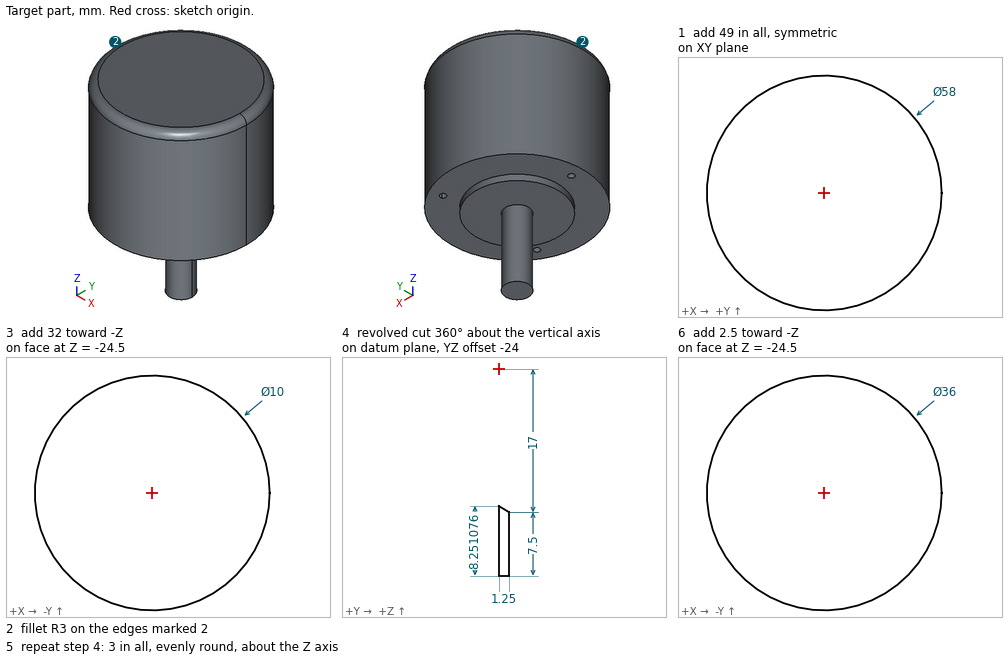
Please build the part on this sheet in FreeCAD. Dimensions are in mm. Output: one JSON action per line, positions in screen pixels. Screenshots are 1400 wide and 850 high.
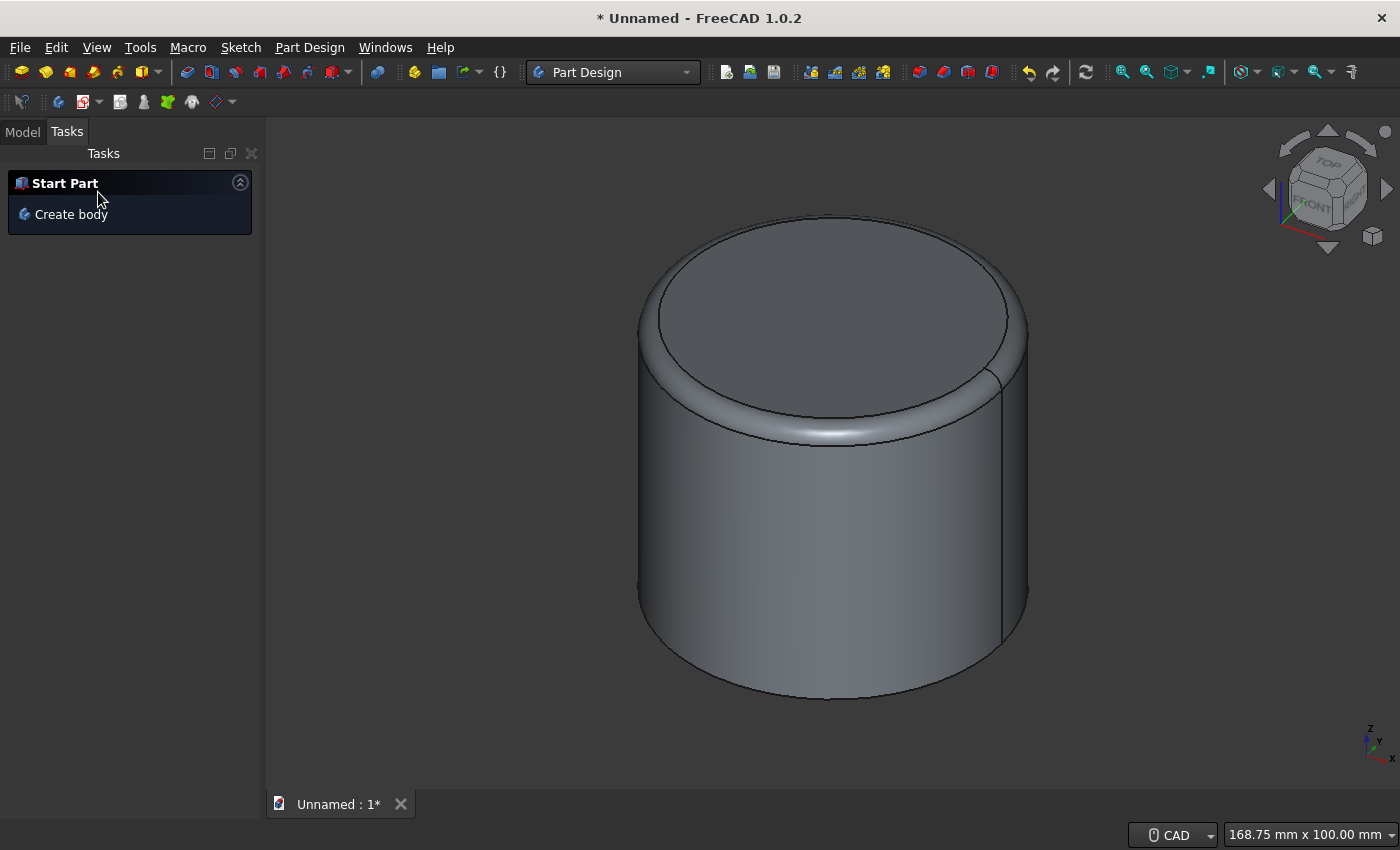
{"action": "key", "text": "5"}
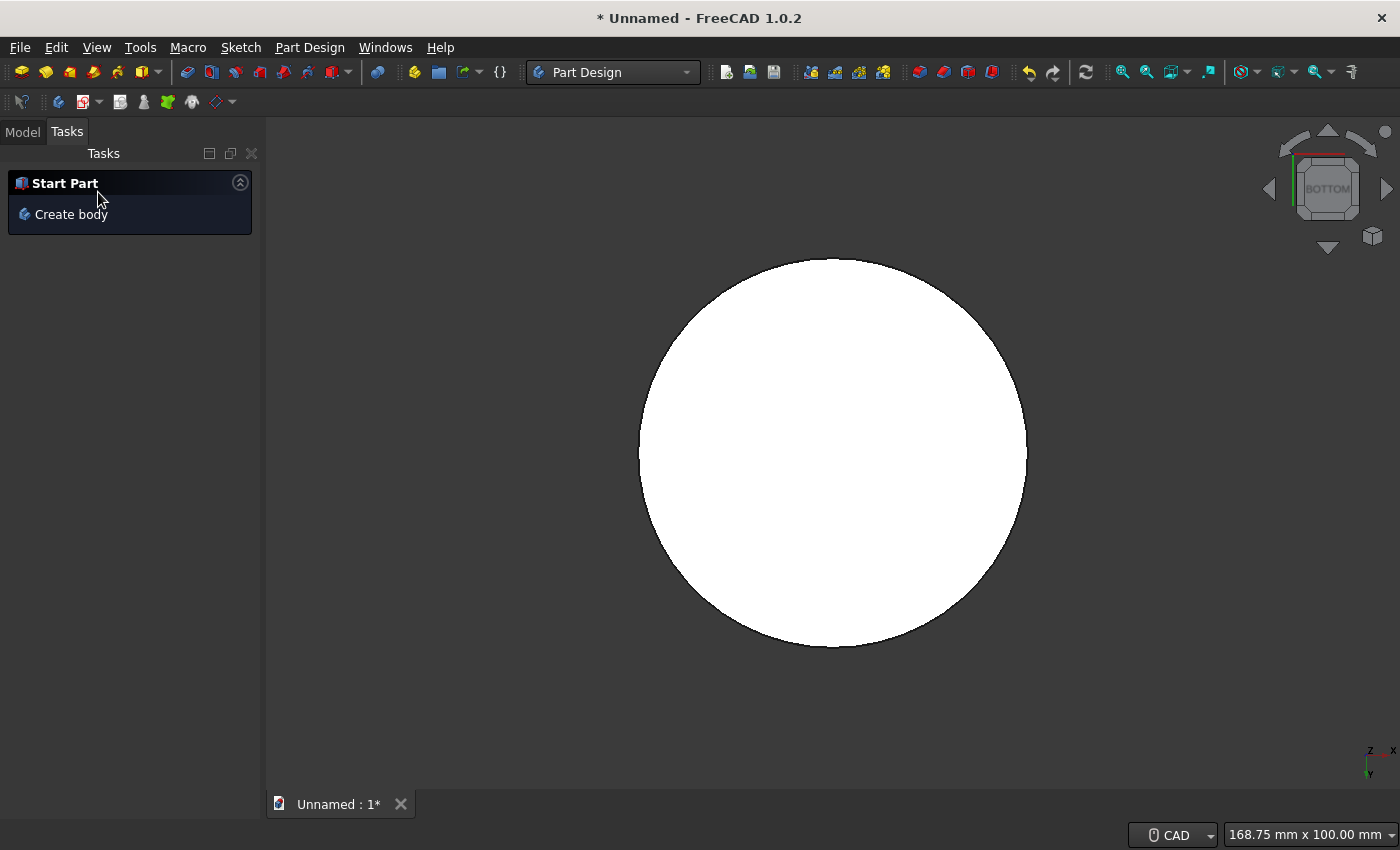
{"action": "left_click", "coordinate": [833, 452]}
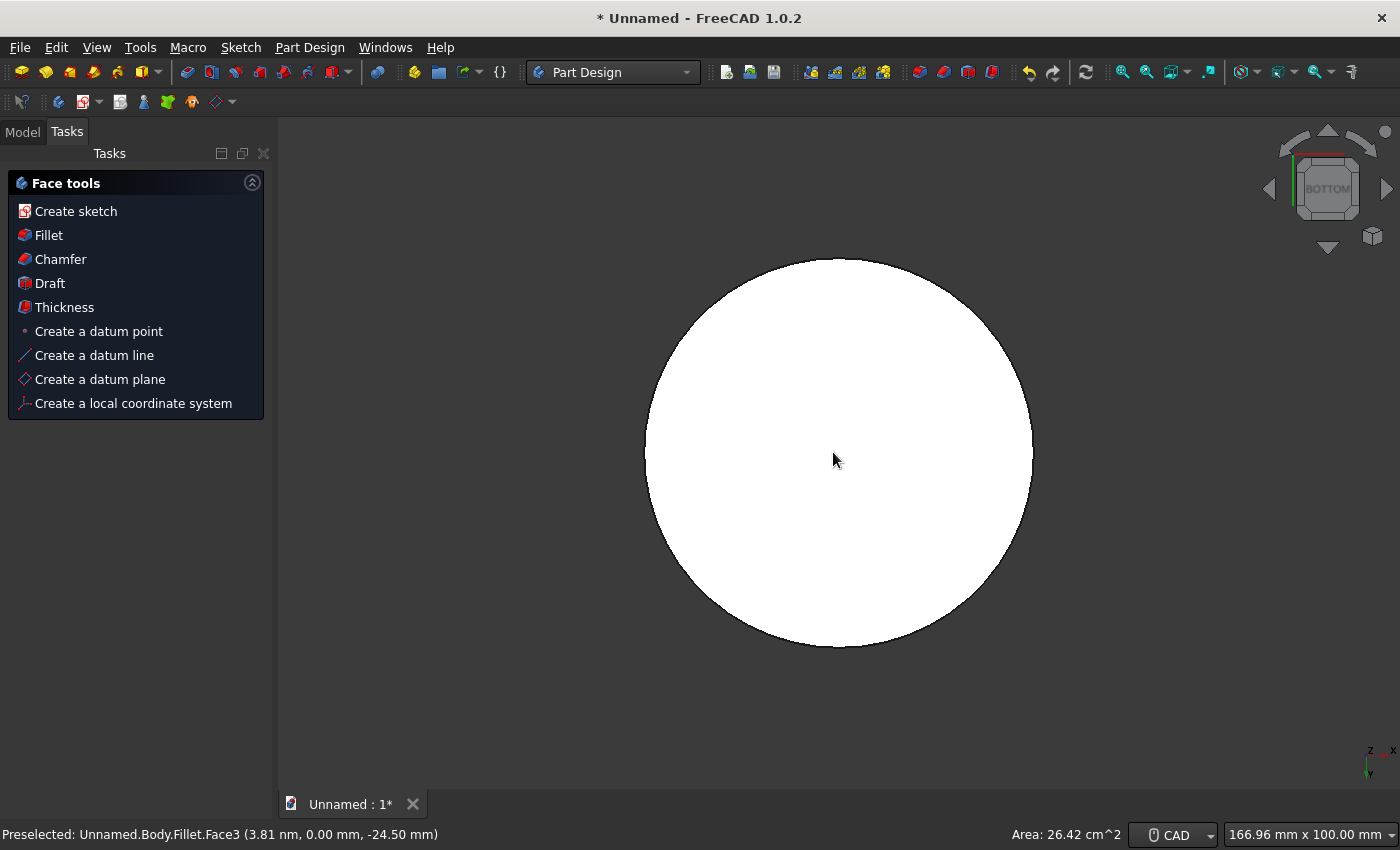
{"action": "left_click", "coordinate": [84, 102]}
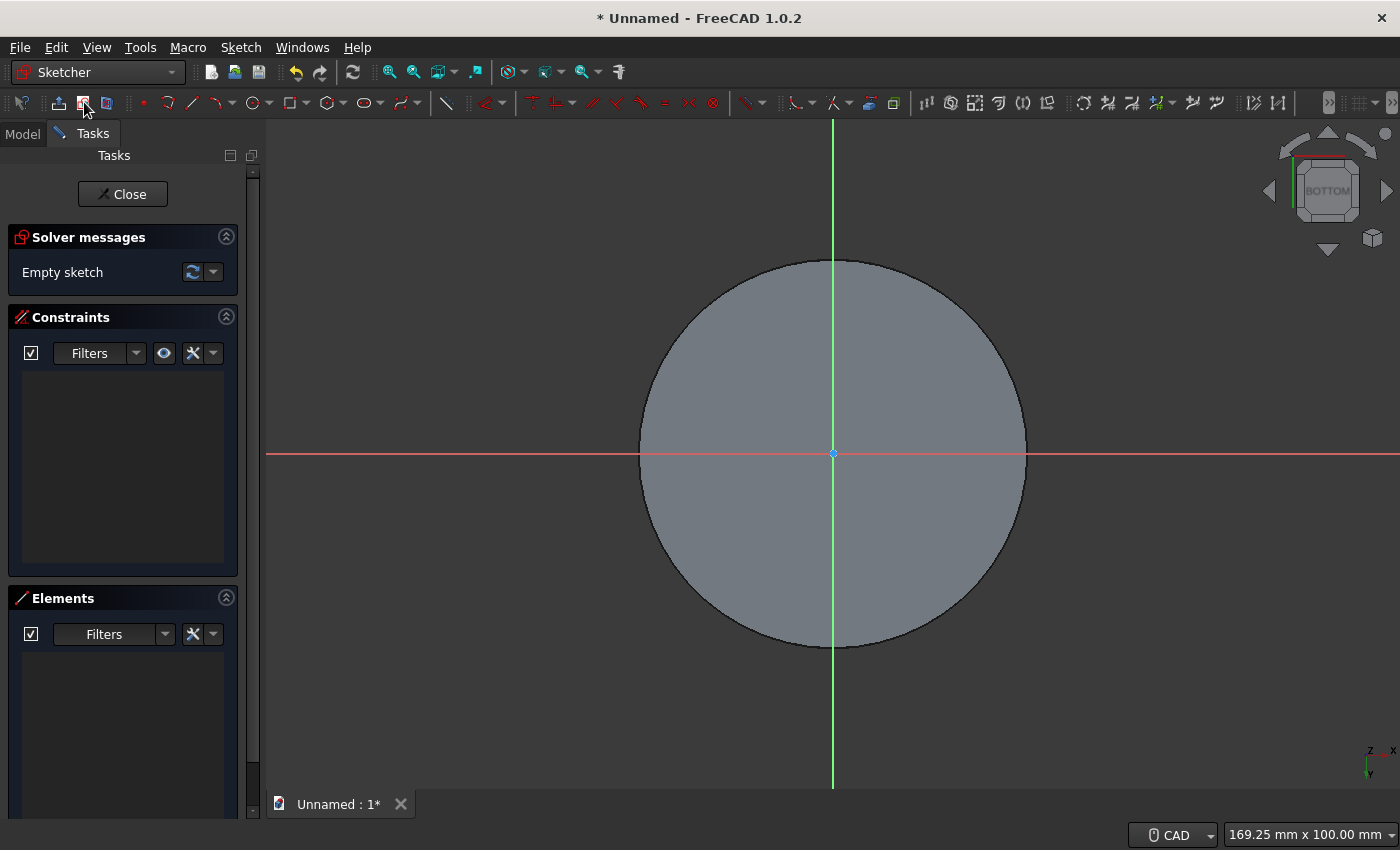
{"action": "scroll", "coordinate": [847, 454], "scroll_direction": "up", "scroll_amount": 9}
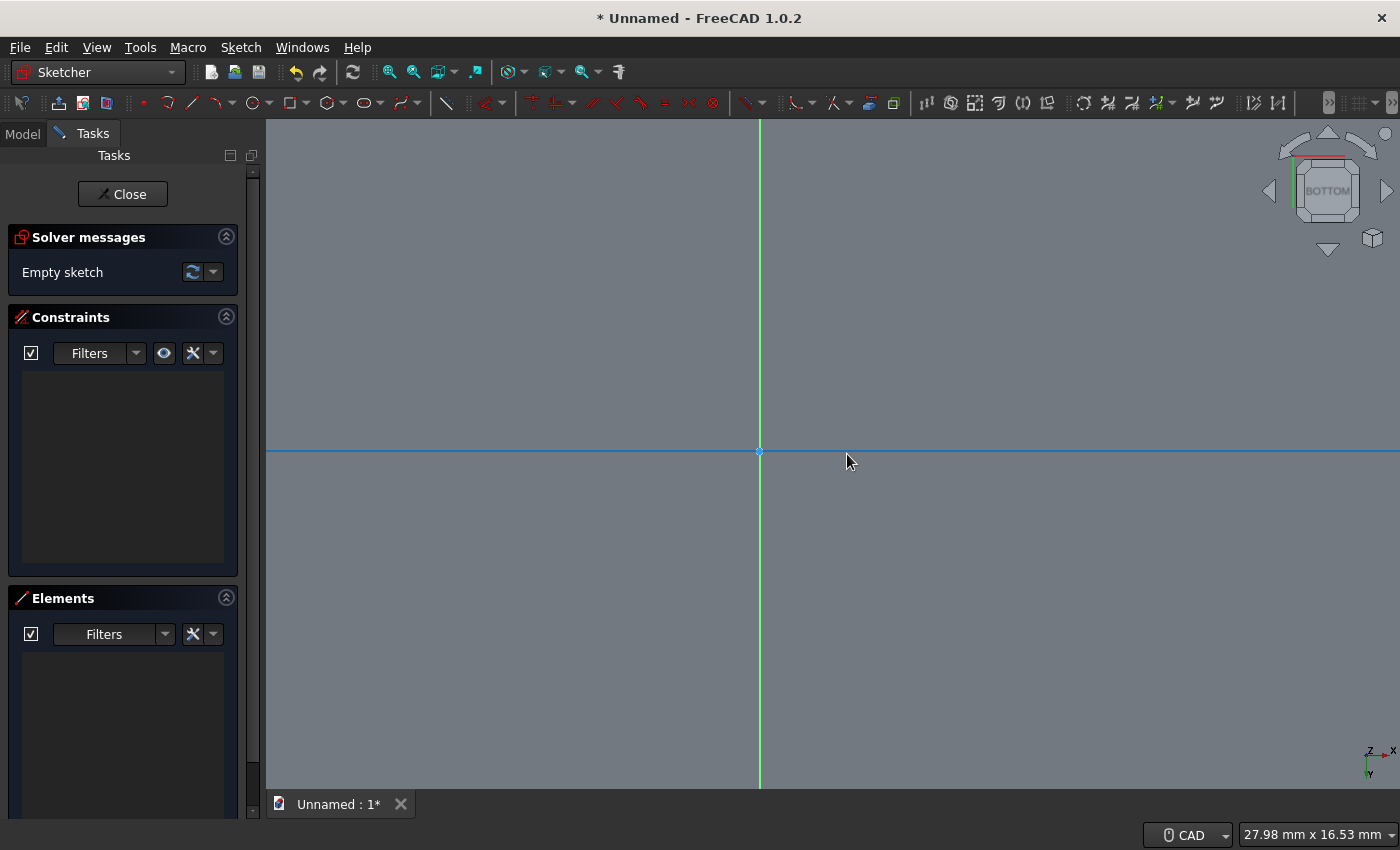
{"action": "left_click", "coordinate": [254, 104]}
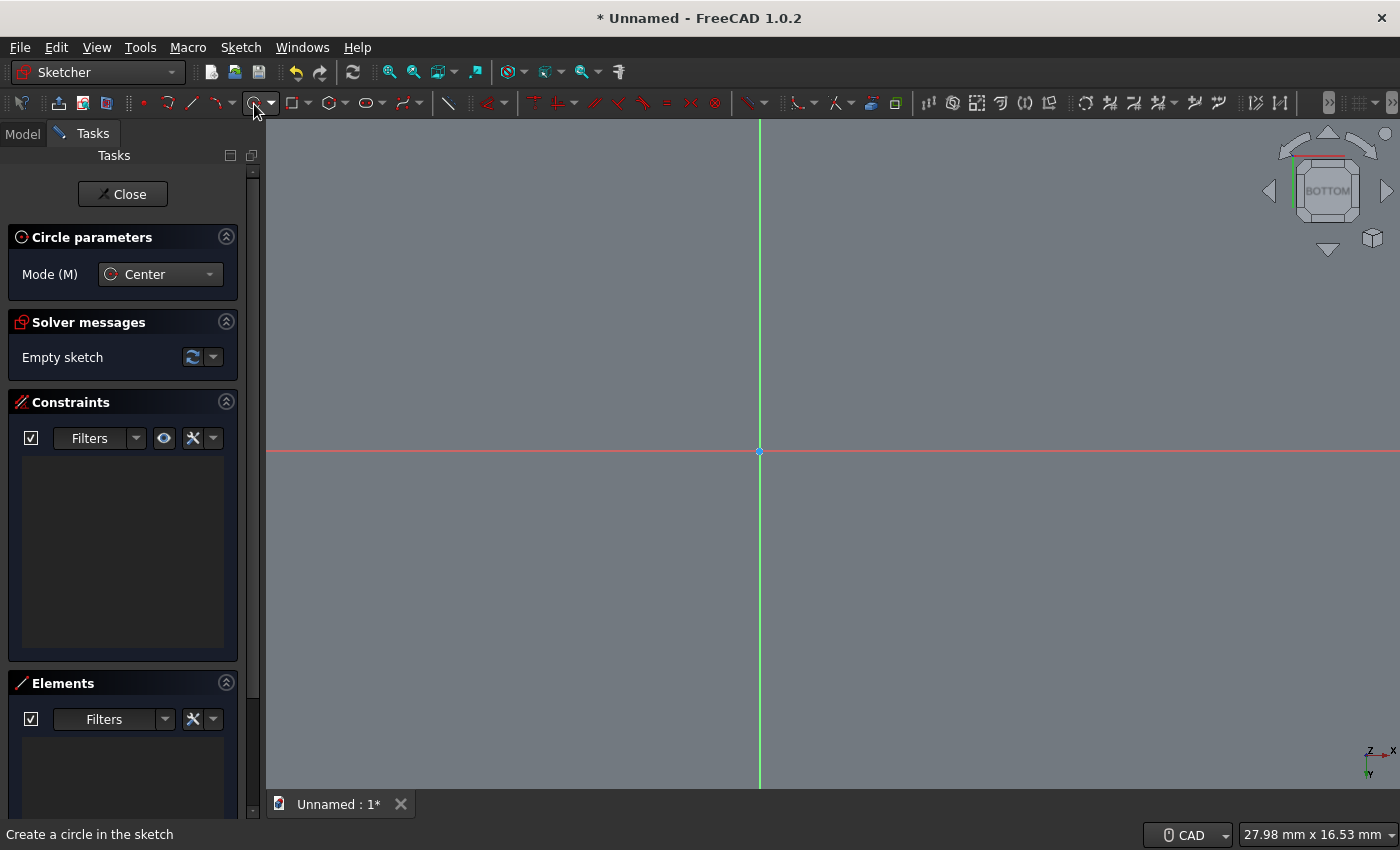
{"action": "left_click", "coordinate": [760, 451]}
{"action": "left_click", "coordinate": [903, 308]}
{"action": "key", "text": "Escape"}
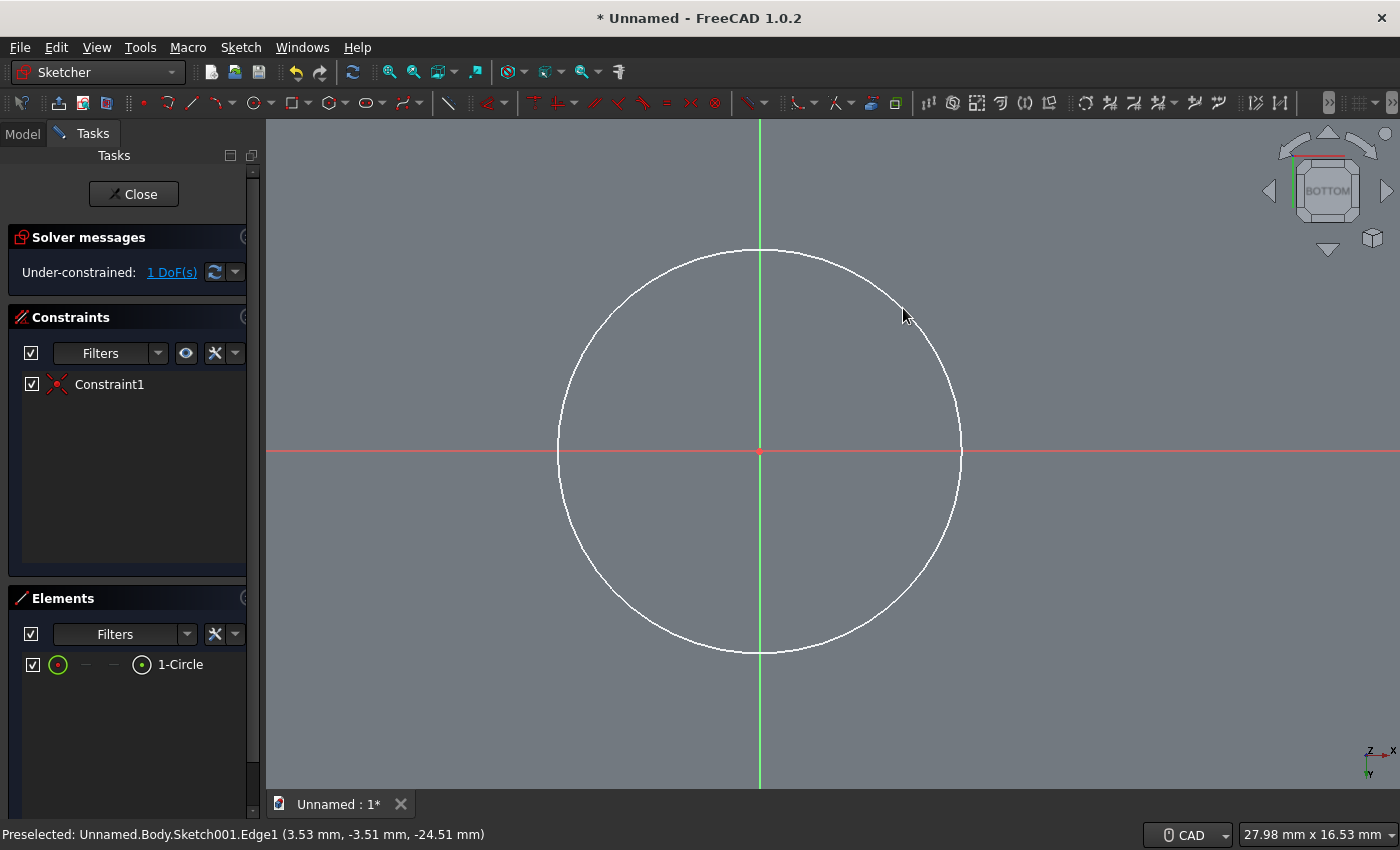
{"action": "left_click", "coordinate": [488, 104]}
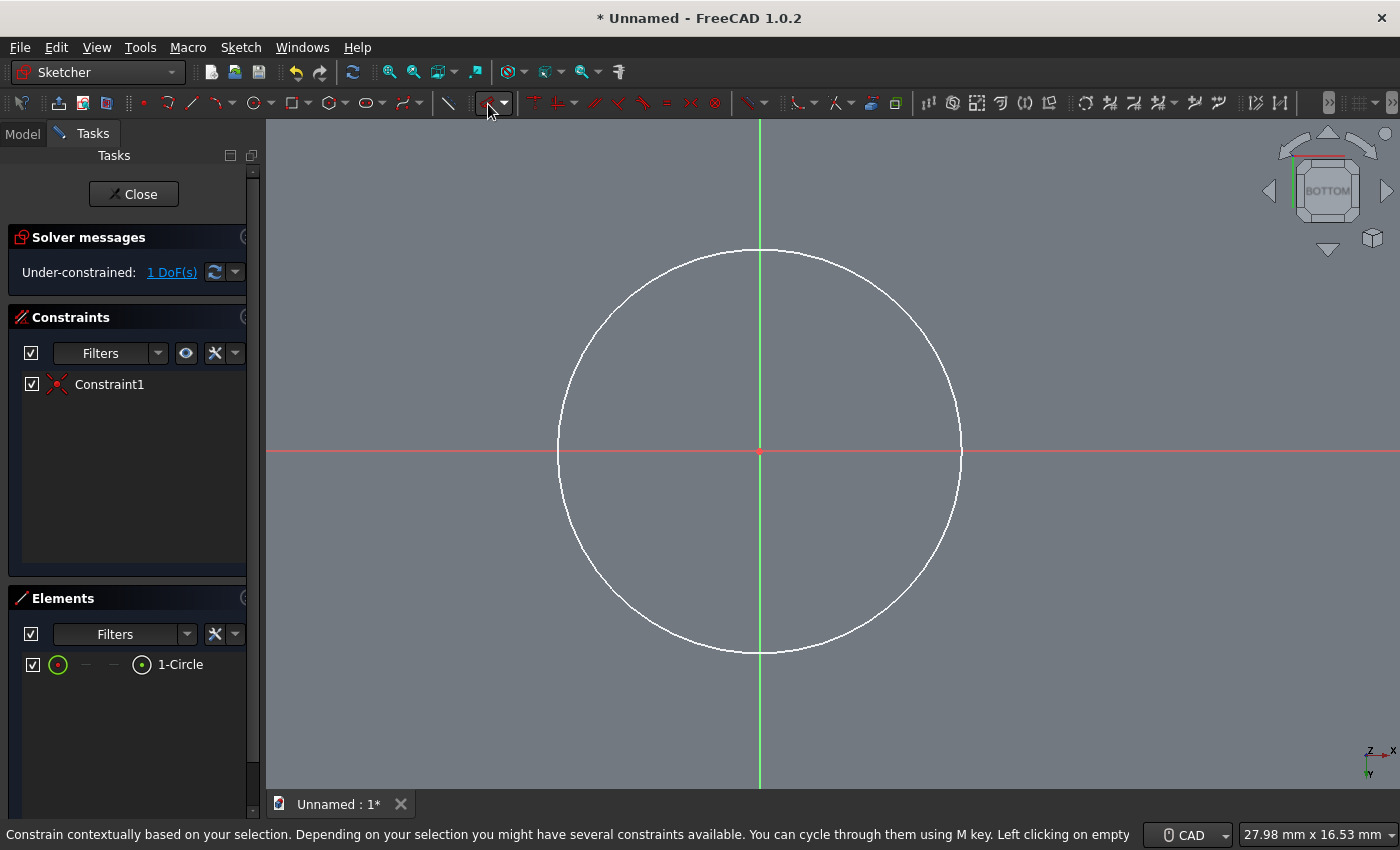
{"action": "left_click", "coordinate": [902, 308]}
{"action": "left_click", "coordinate": [925, 285]}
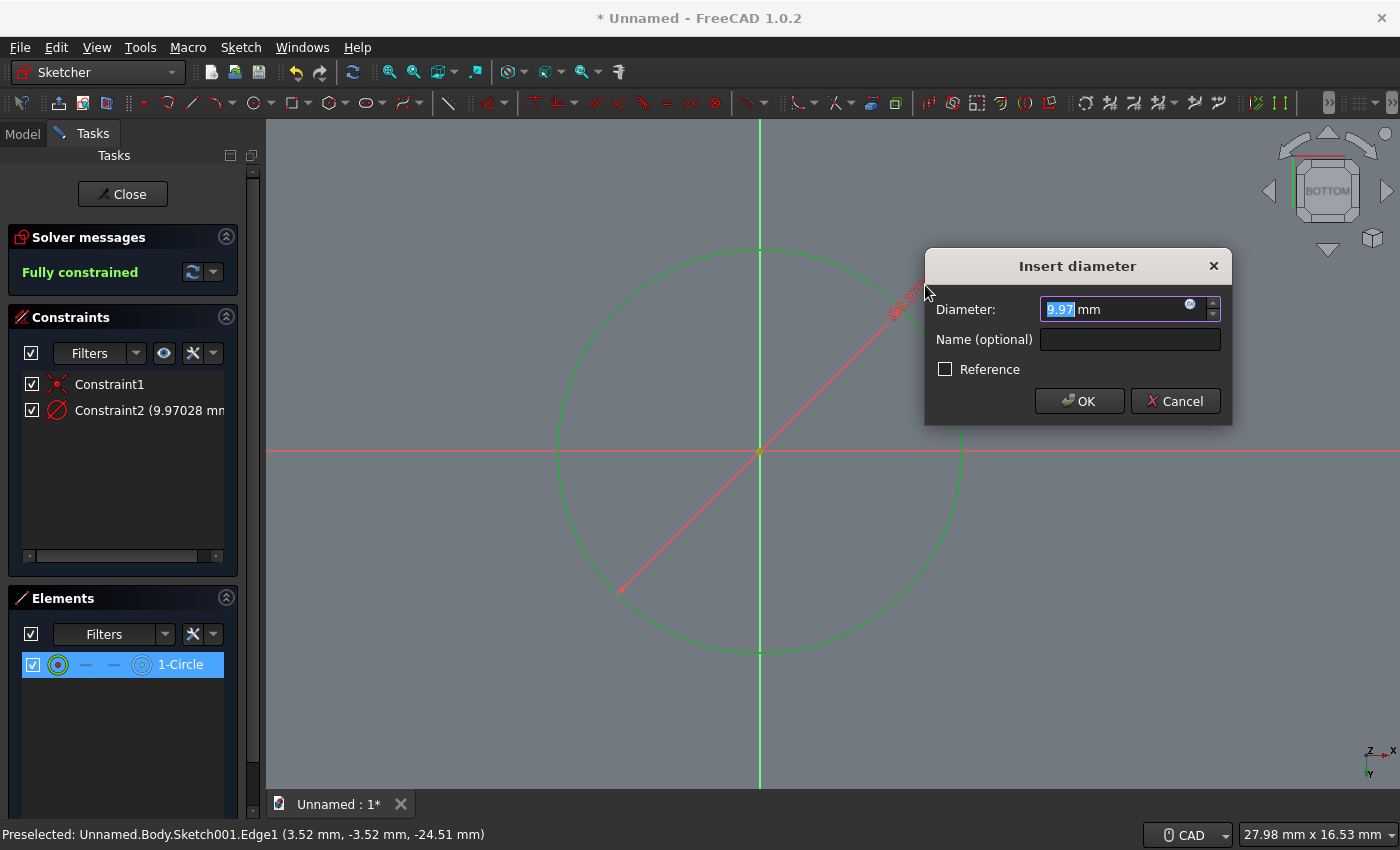
{"action": "type", "text": "10"}
{"action": "key", "text": "Return"}
{"action": "key", "text": "Escape"}